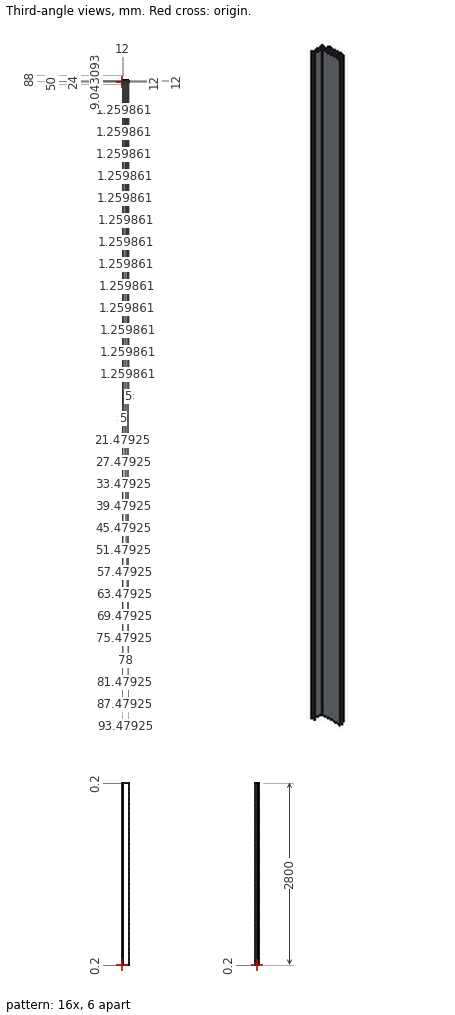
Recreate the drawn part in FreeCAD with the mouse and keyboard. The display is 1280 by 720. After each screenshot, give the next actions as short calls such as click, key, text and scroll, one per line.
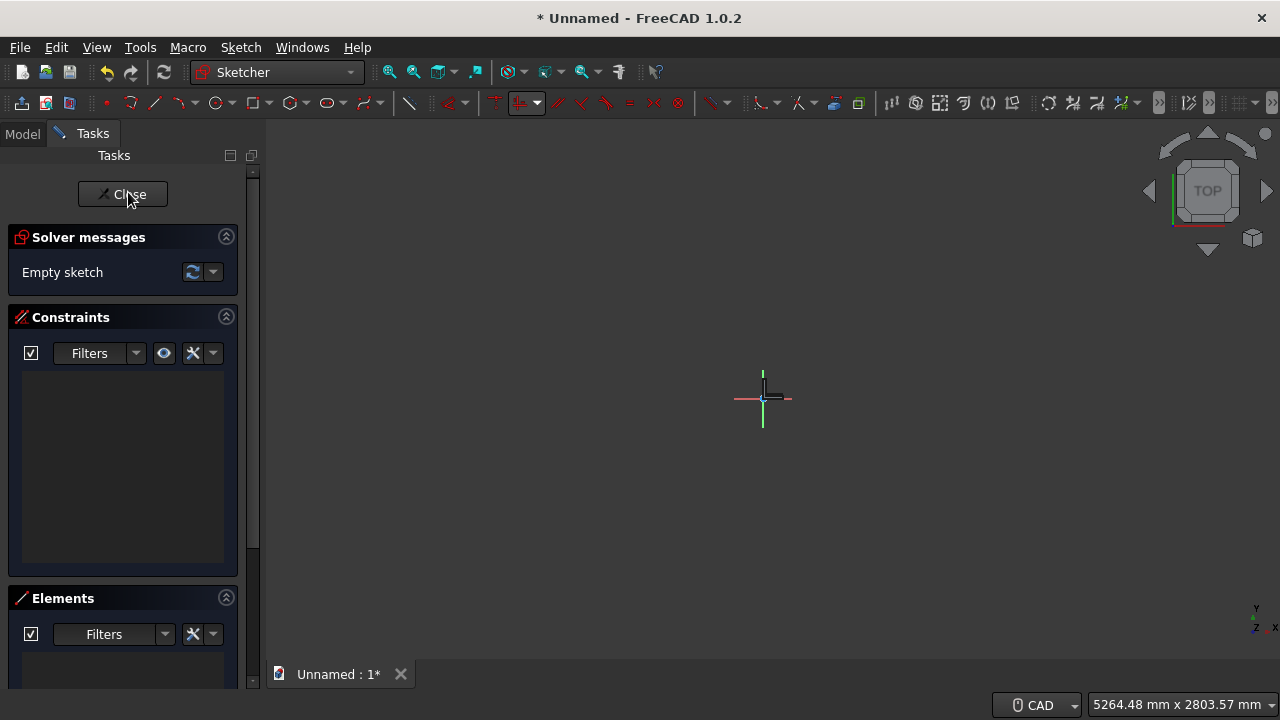
click(70, 104)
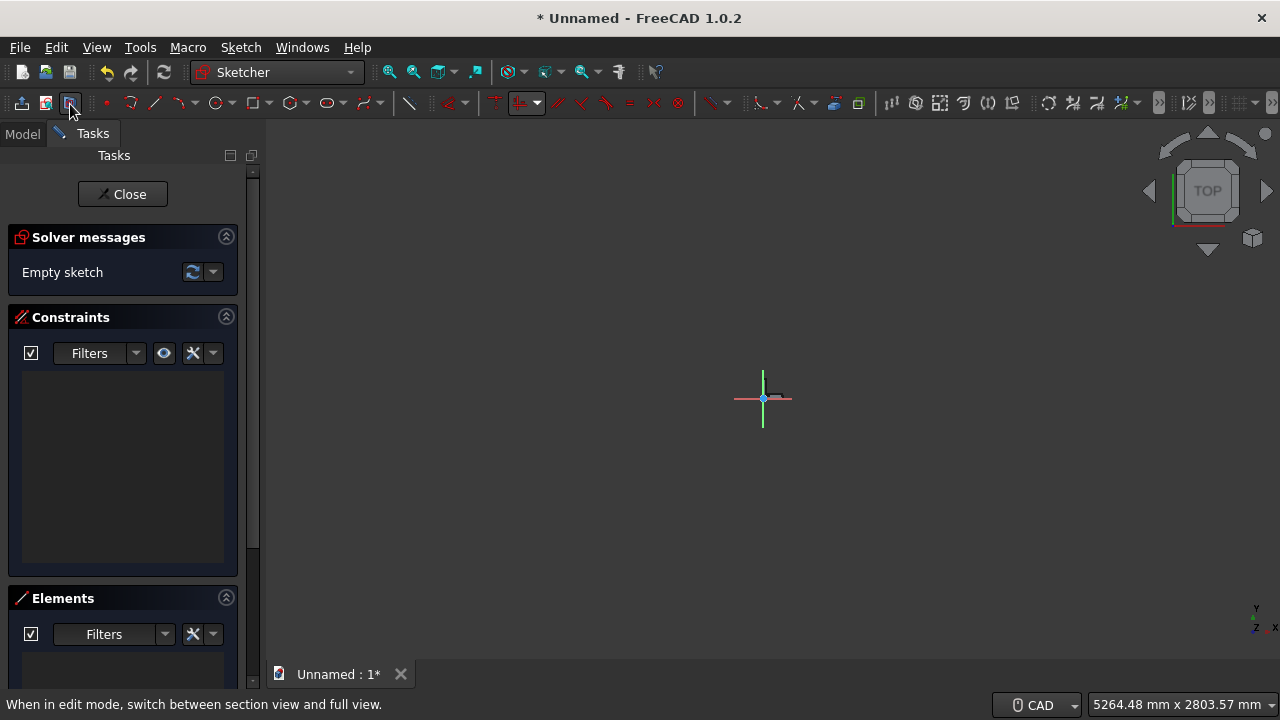
scroll(773, 395, up, 15)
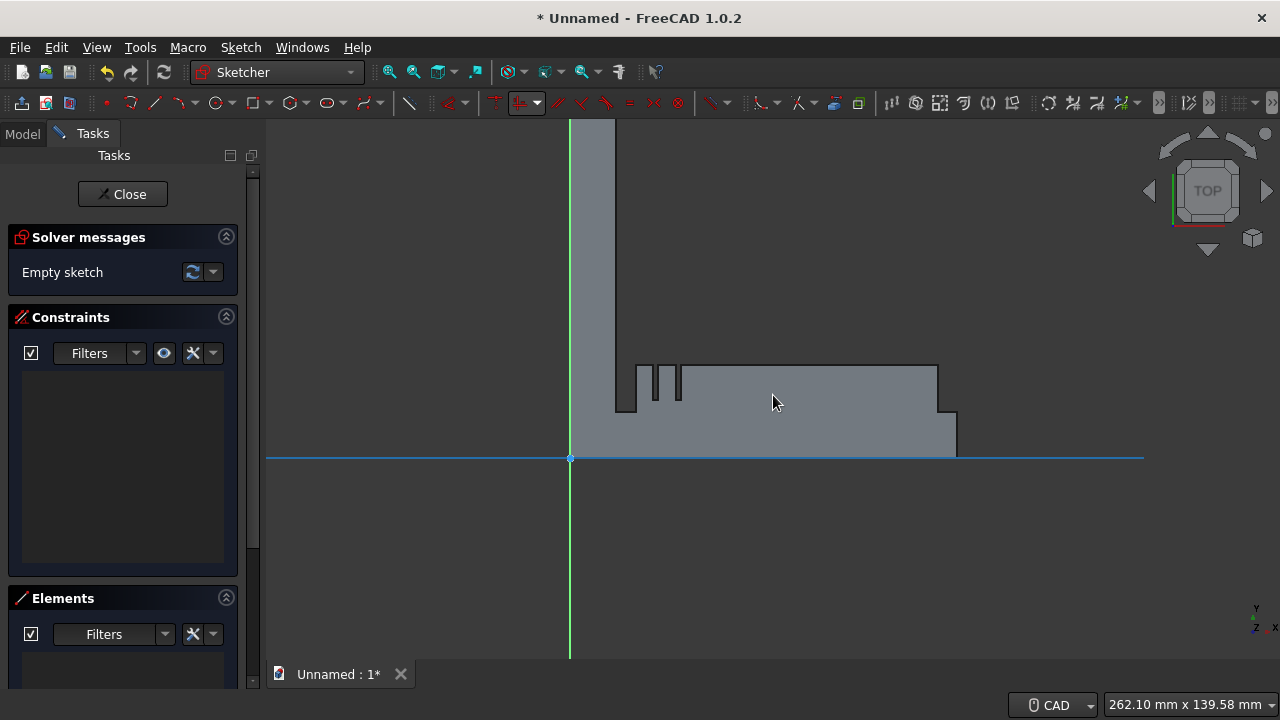
scroll(702, 382, up, 11)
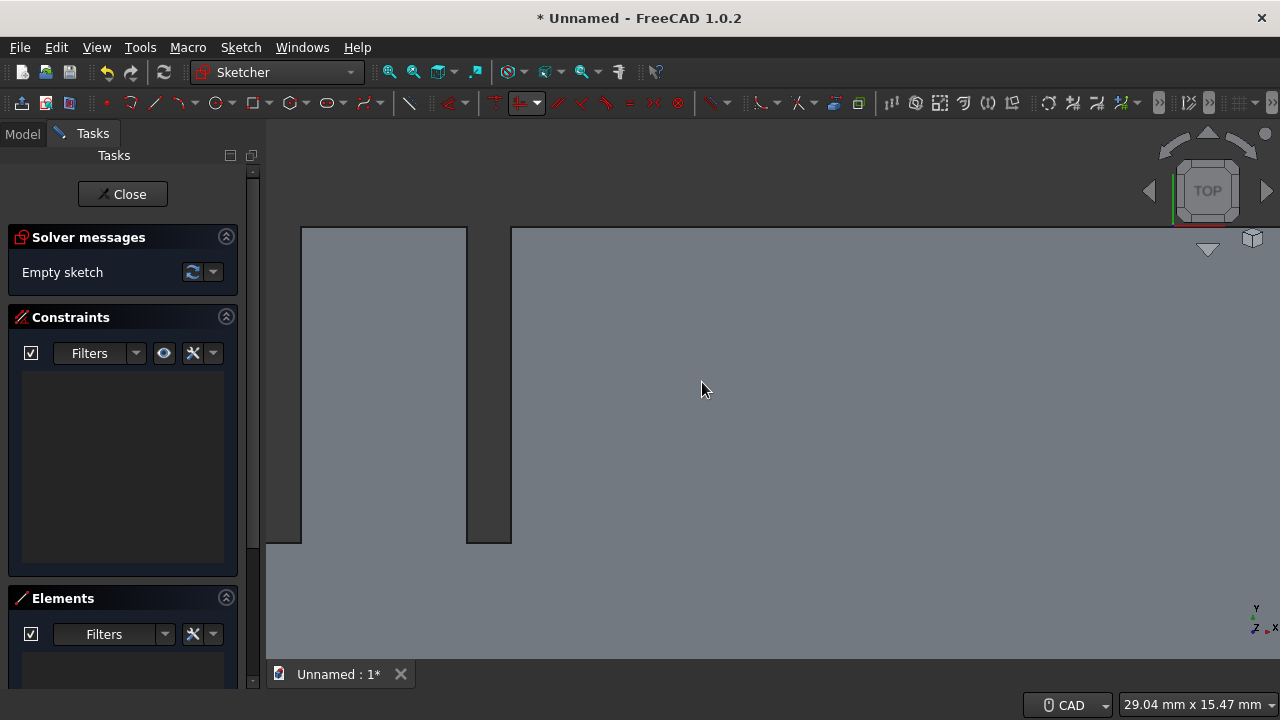
click(254, 104)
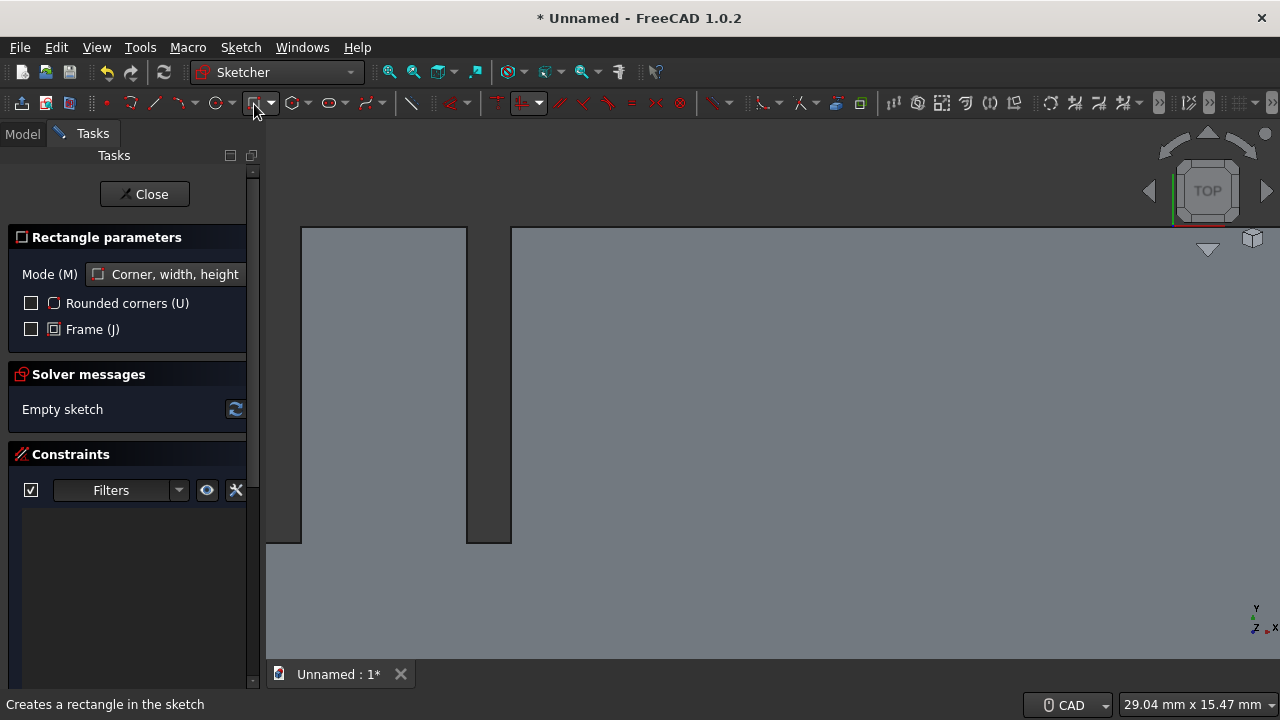
click(676, 227)
move(720, 543)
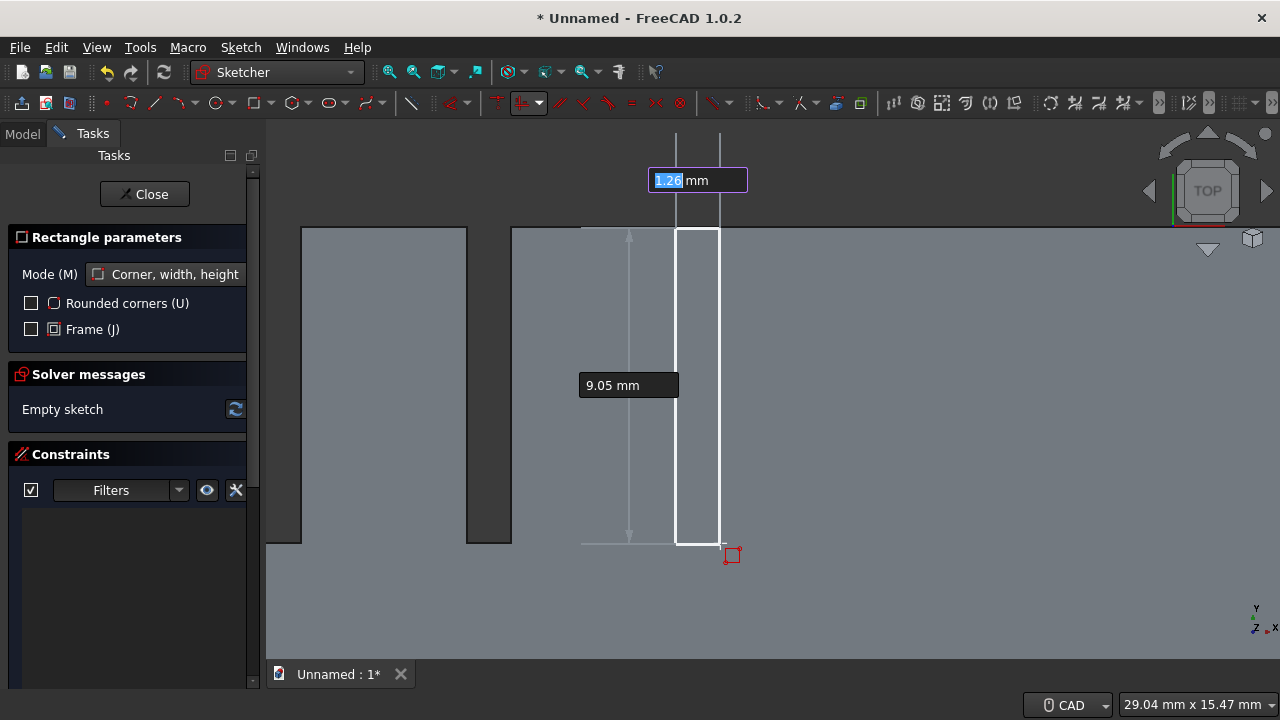
text(1.259861)
key(Tab)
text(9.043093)
key(Return)
key(Escape)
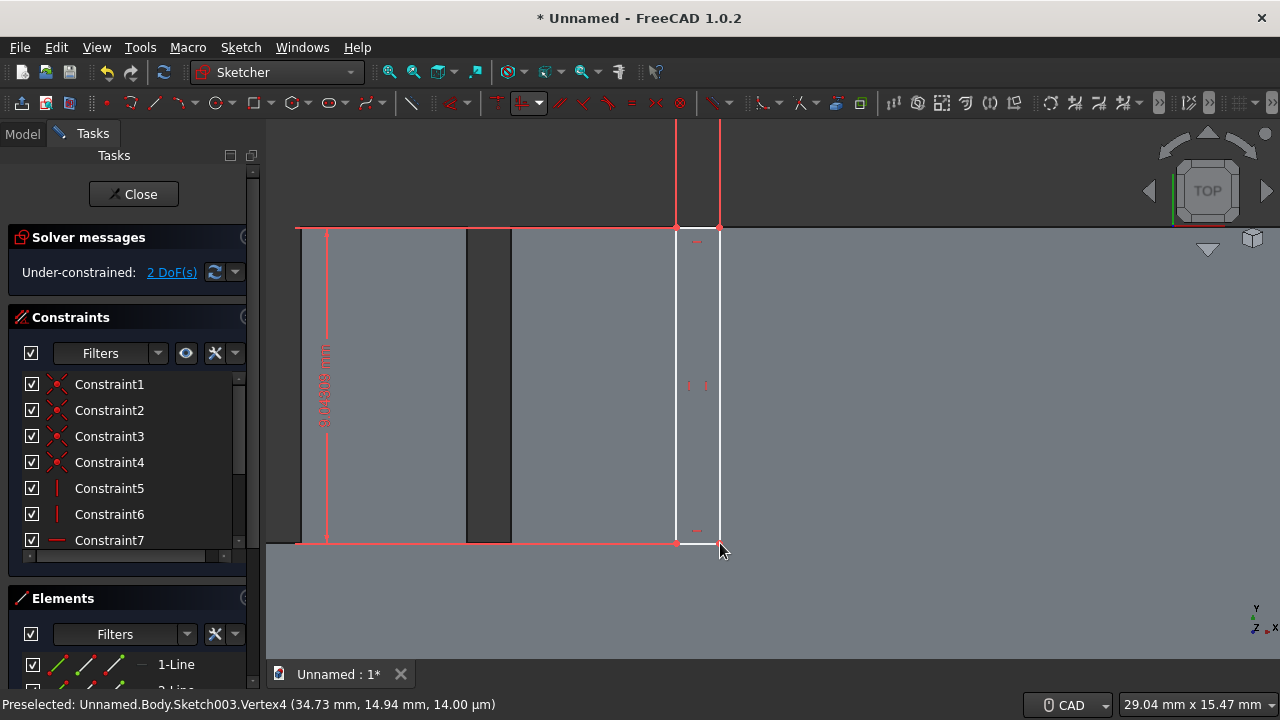
click(450, 104)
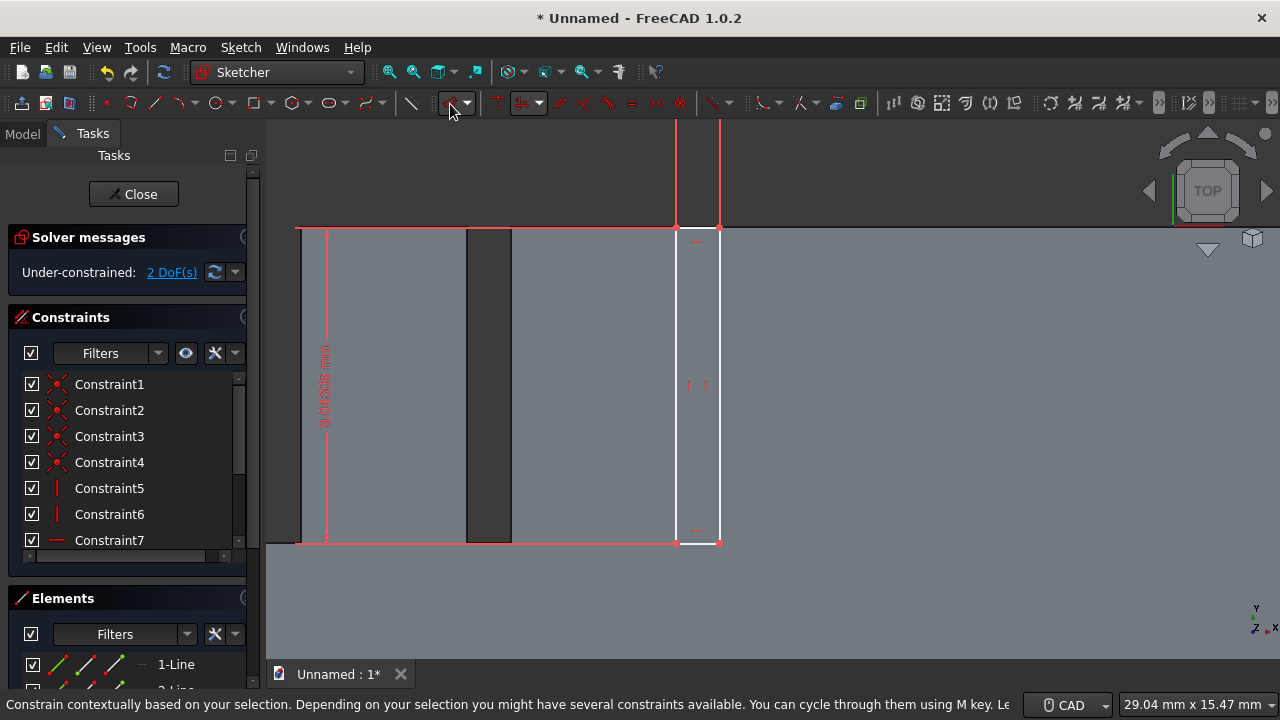
click(676, 228)
click(710, 571)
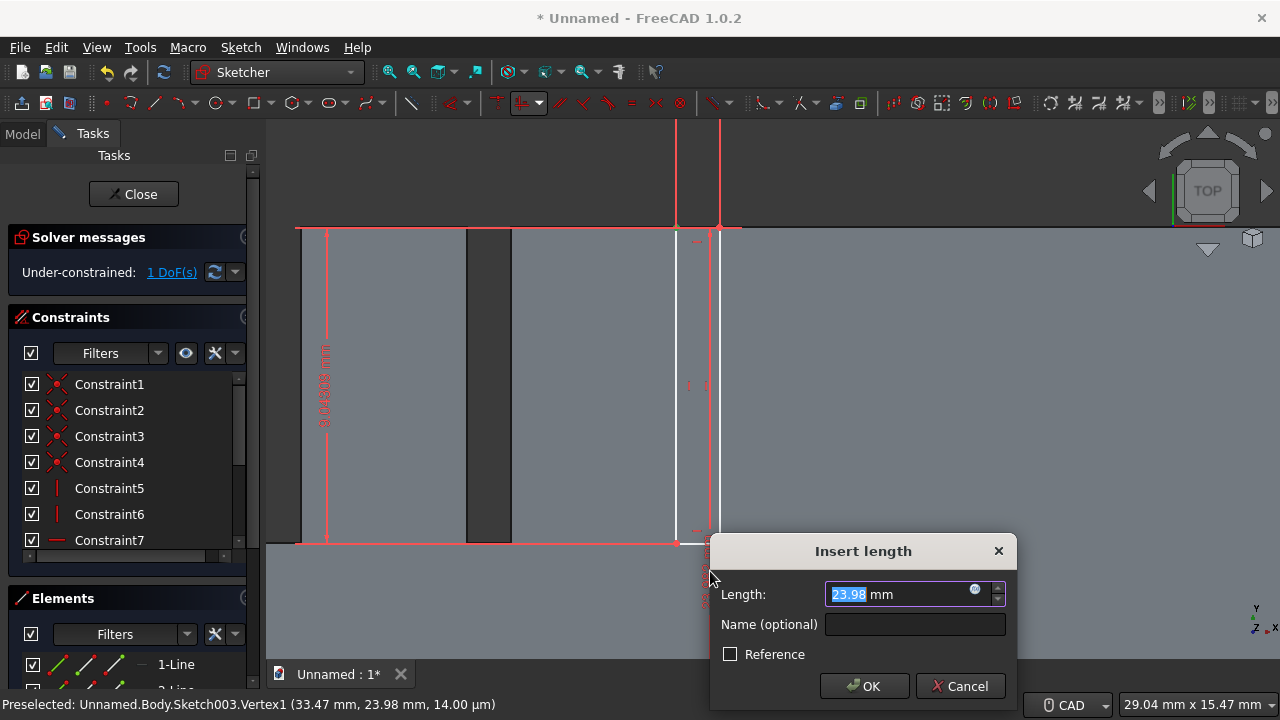
text(24)
key(Return)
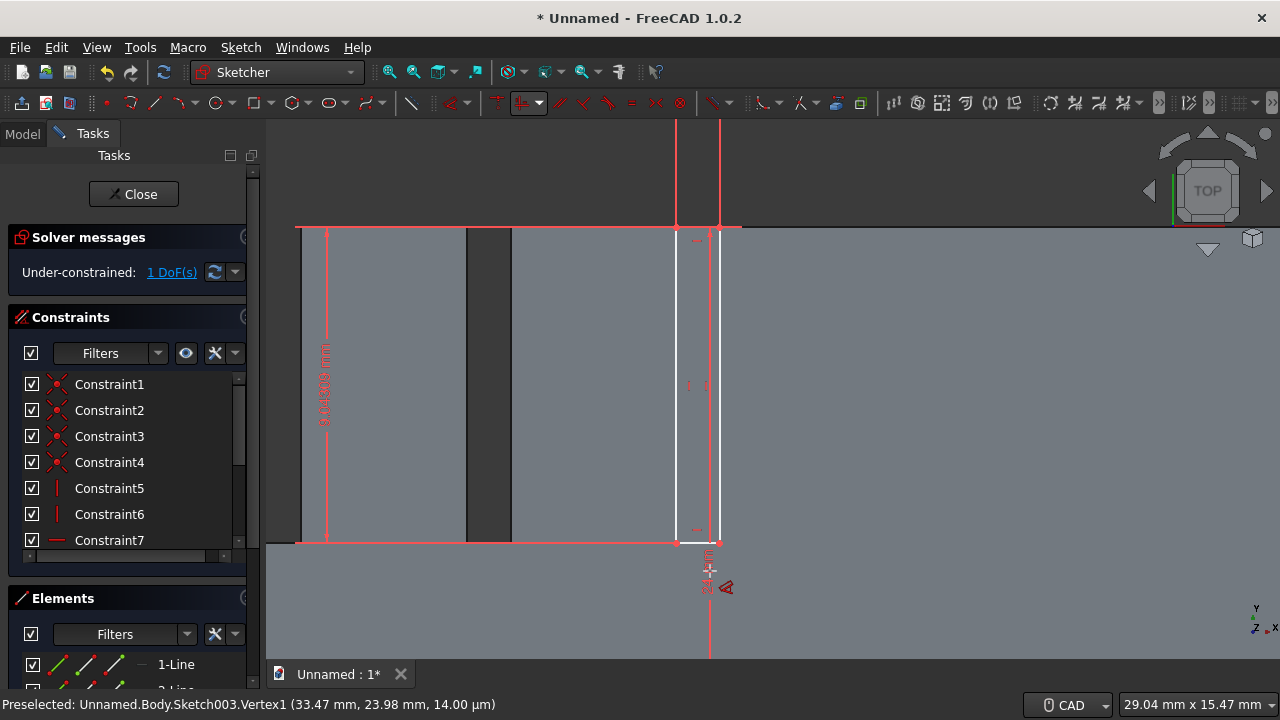
click(676, 227)
click(485, 193)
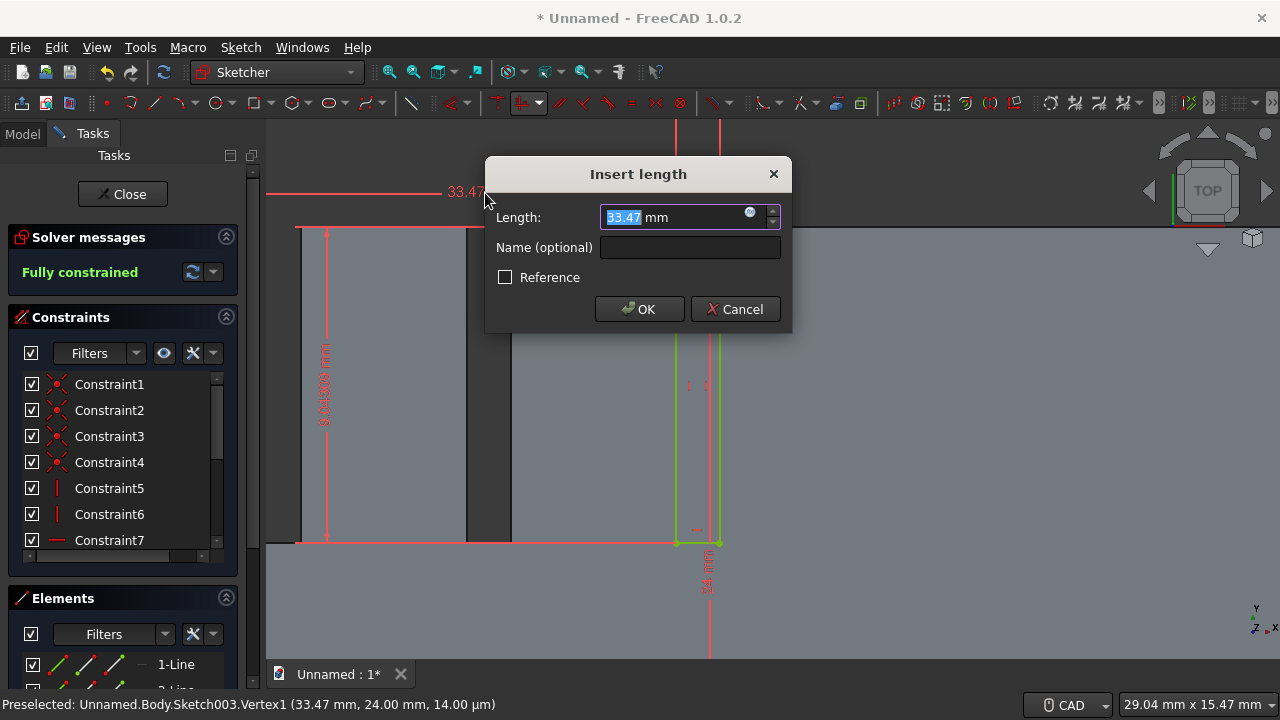
text(33.47925)
key(Return)
key(Escape)